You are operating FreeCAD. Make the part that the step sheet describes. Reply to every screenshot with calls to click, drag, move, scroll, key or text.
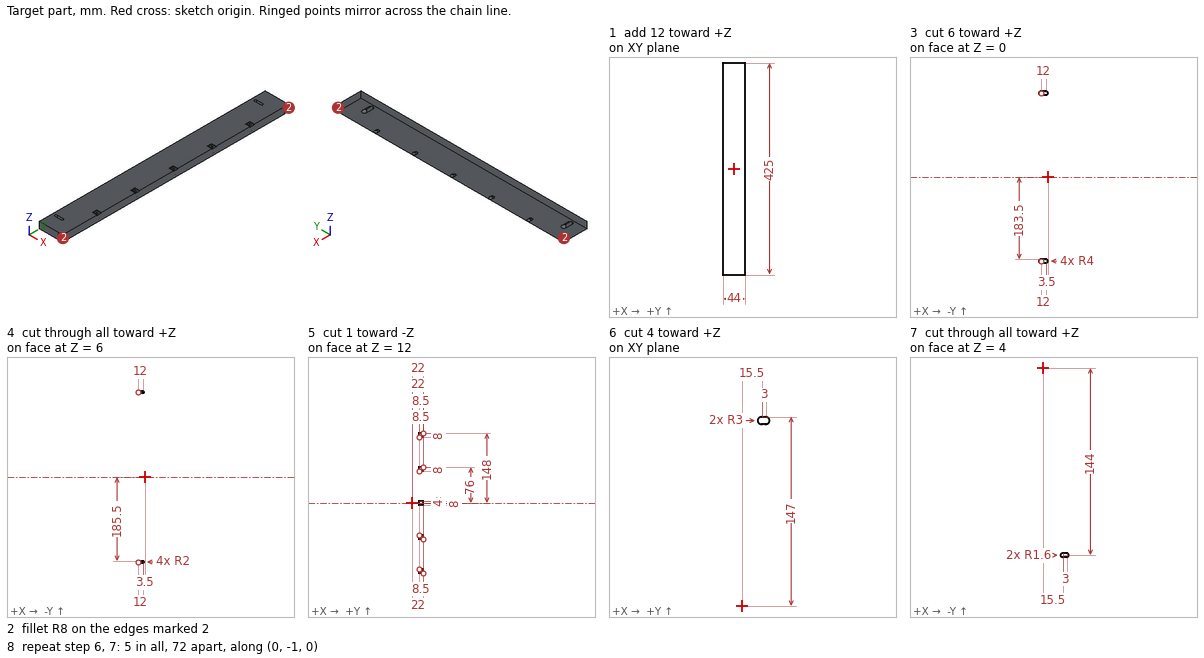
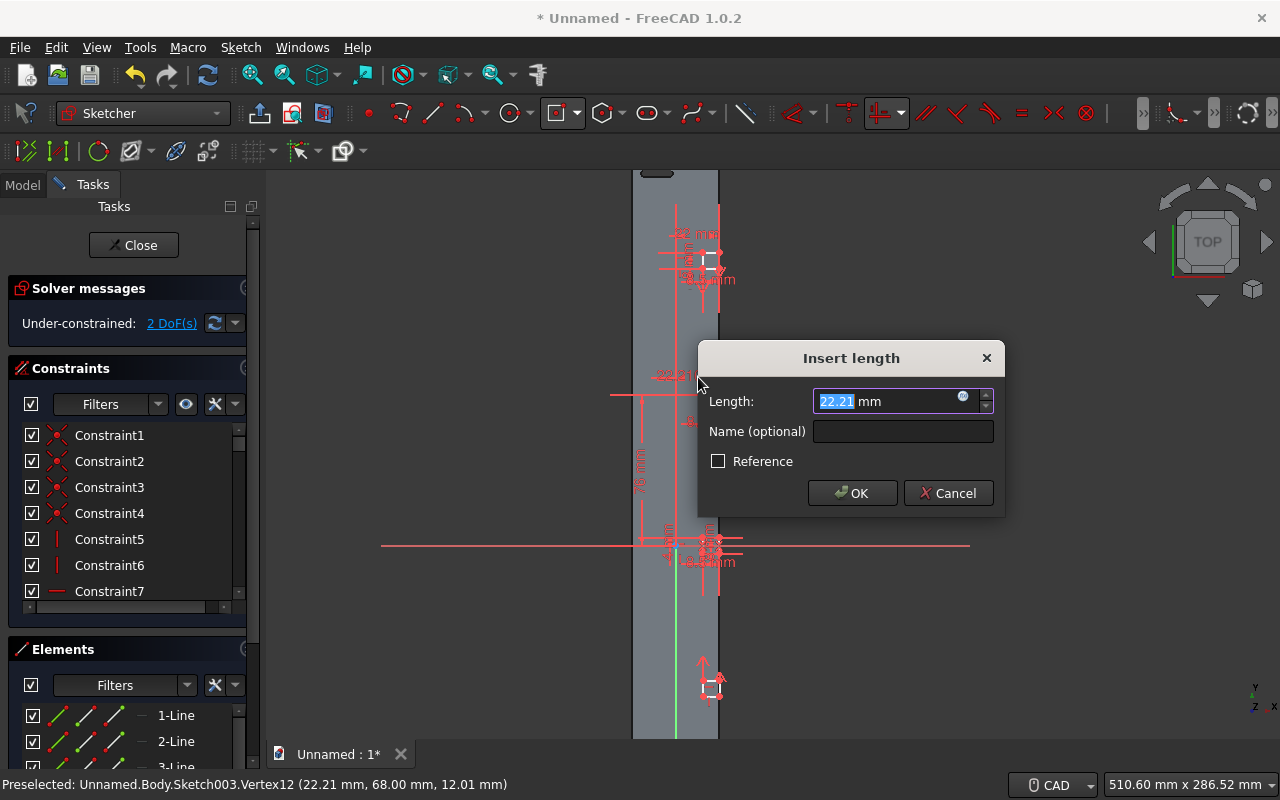
text(22)
key(Return)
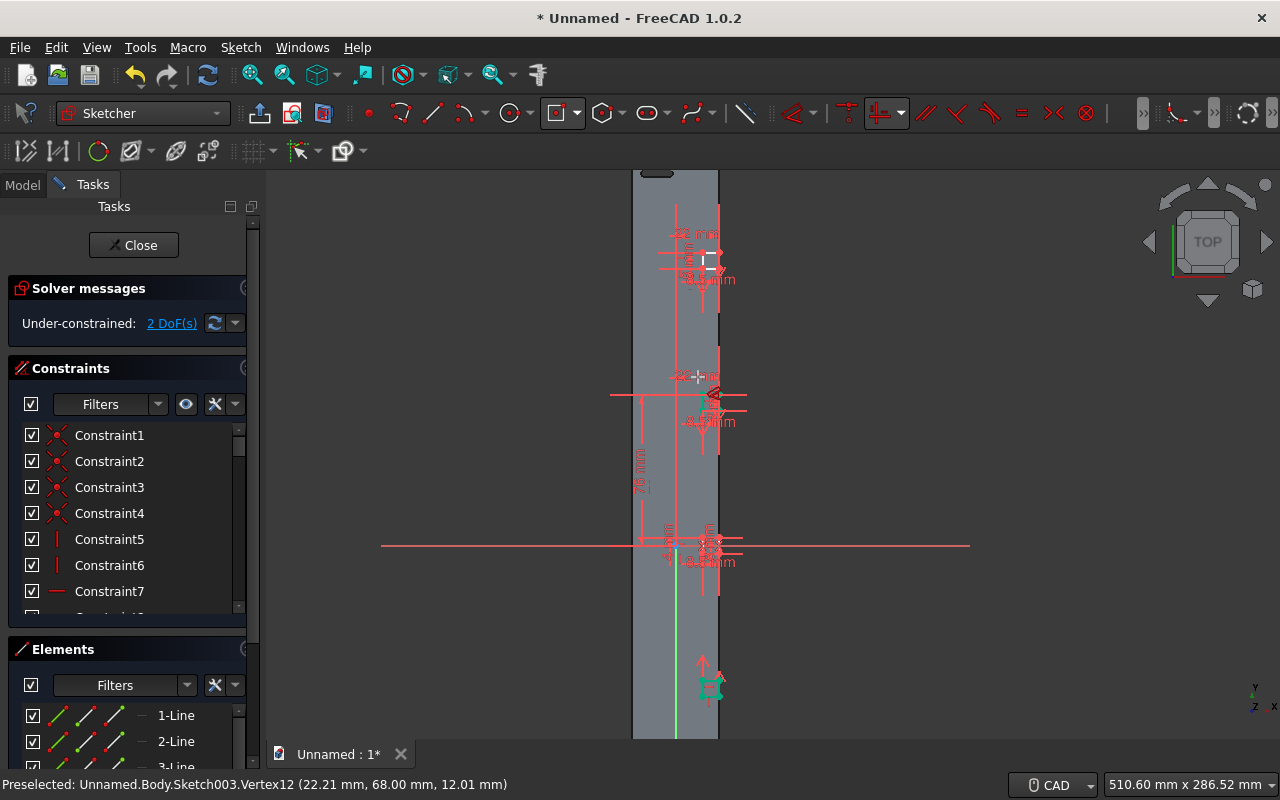
click(719, 554)
click(698, 588)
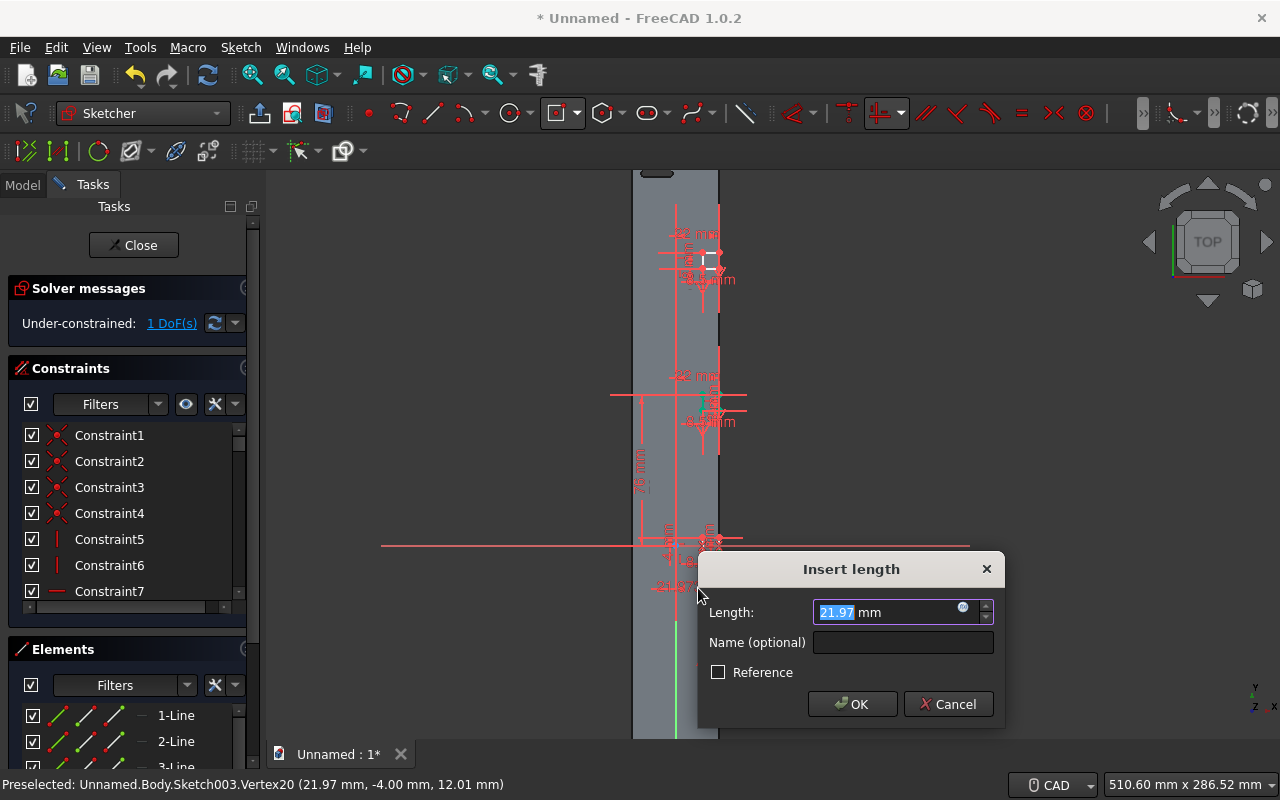
text(22)
key(Return)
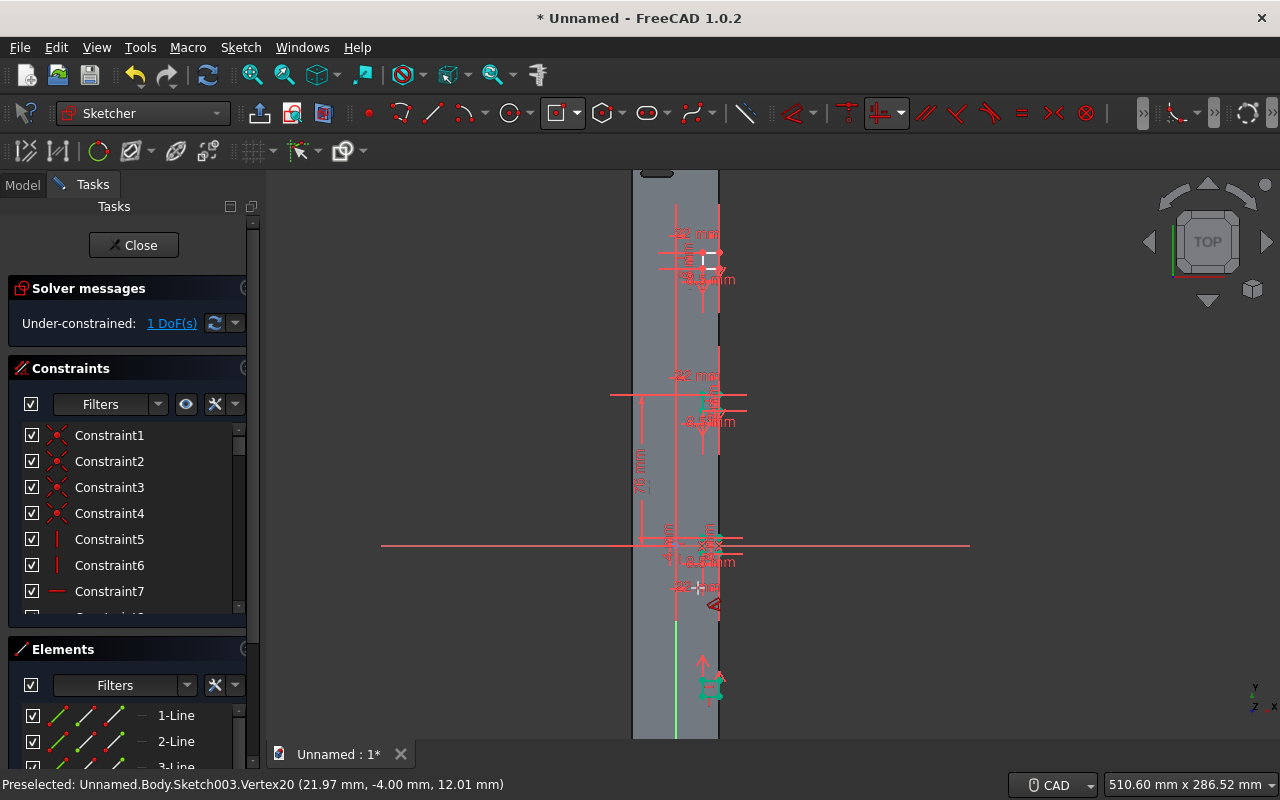
click(703, 253)
click(642, 399)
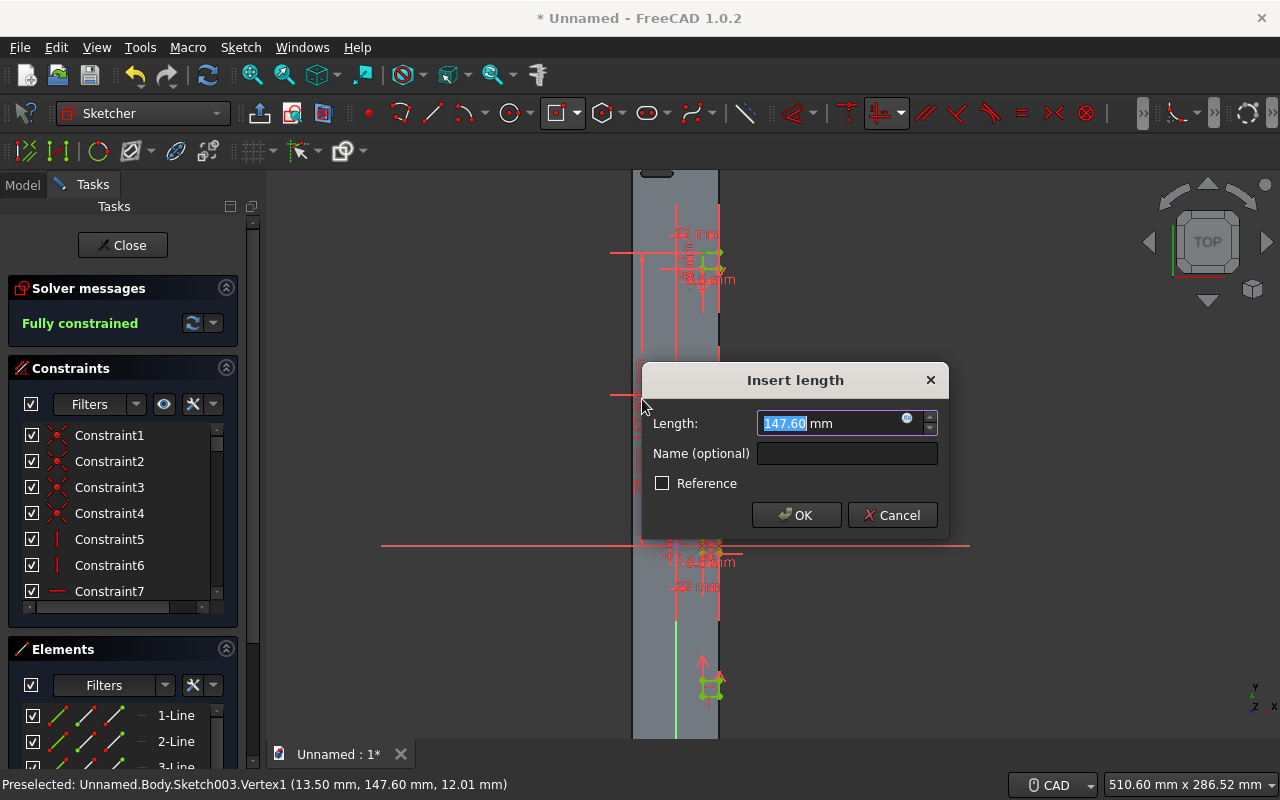
text(148)
key(Return)
key(Escape)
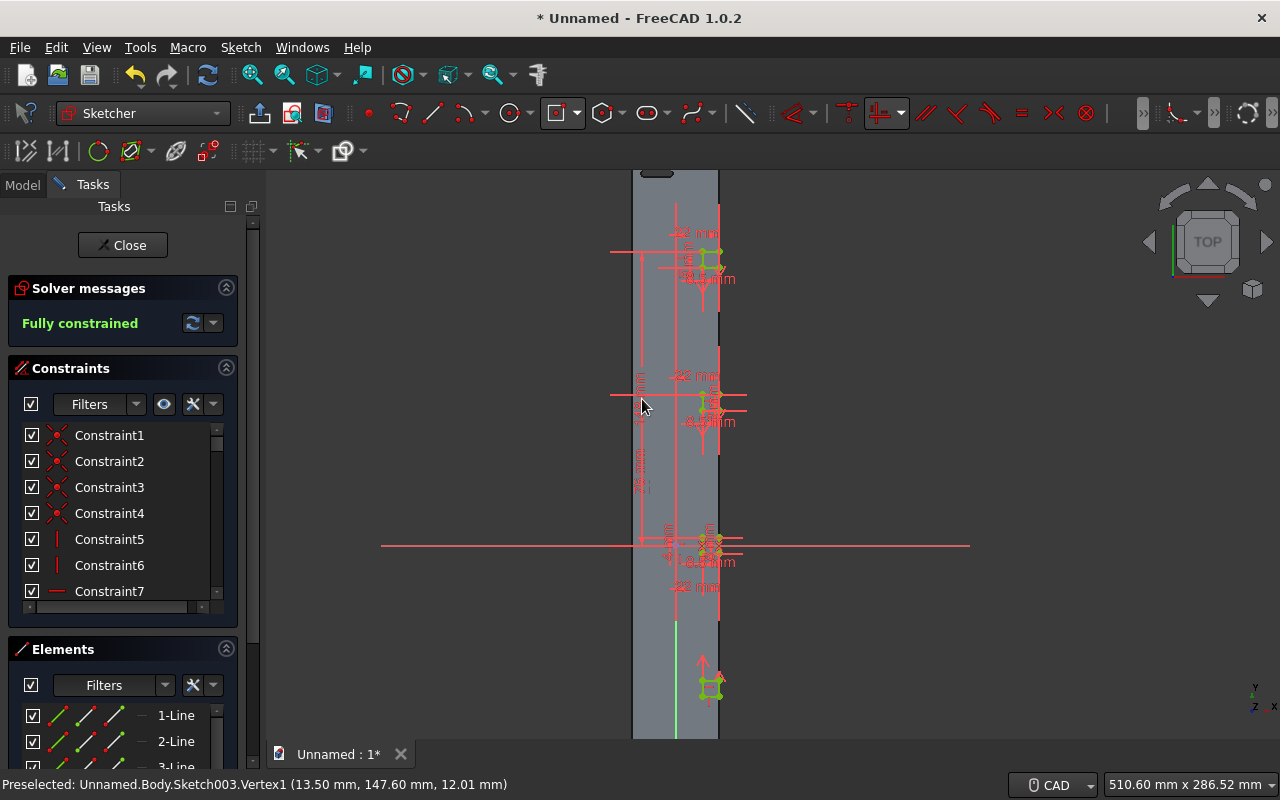
click(123, 245)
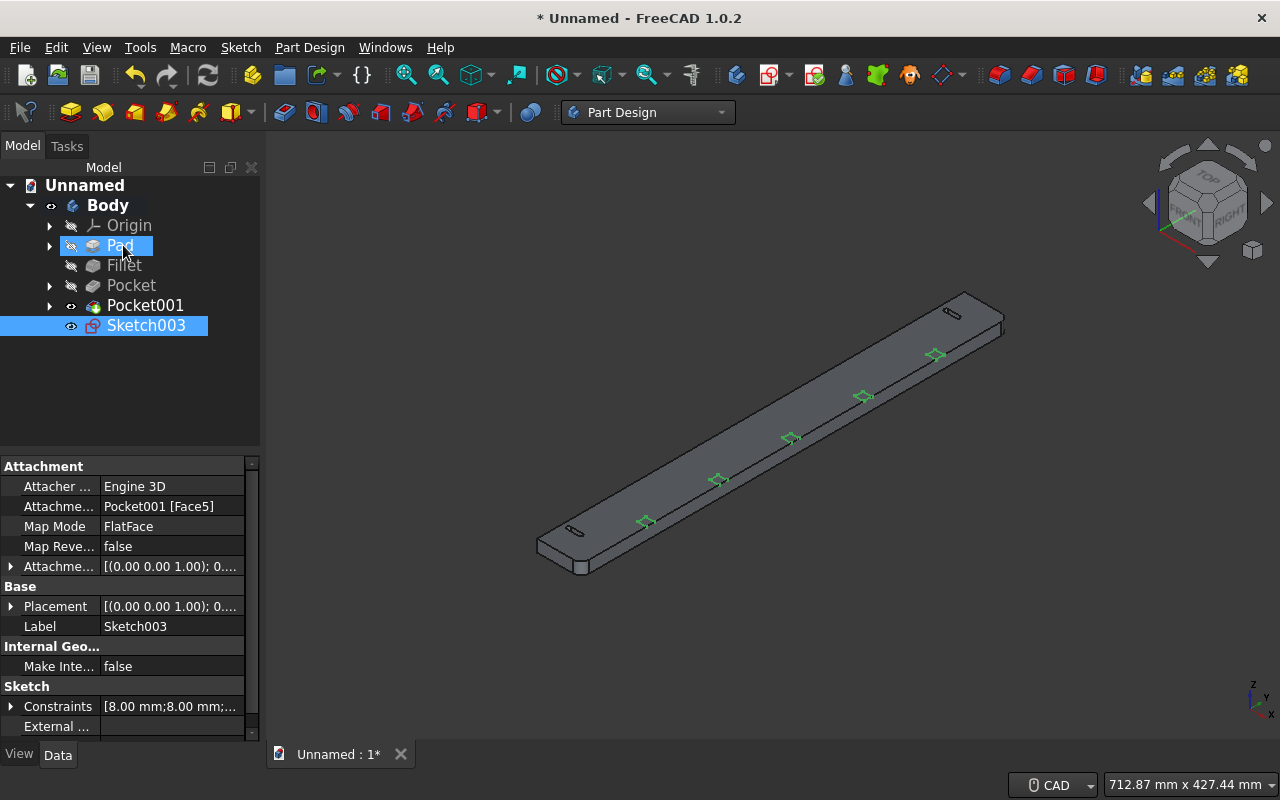
click(286, 112)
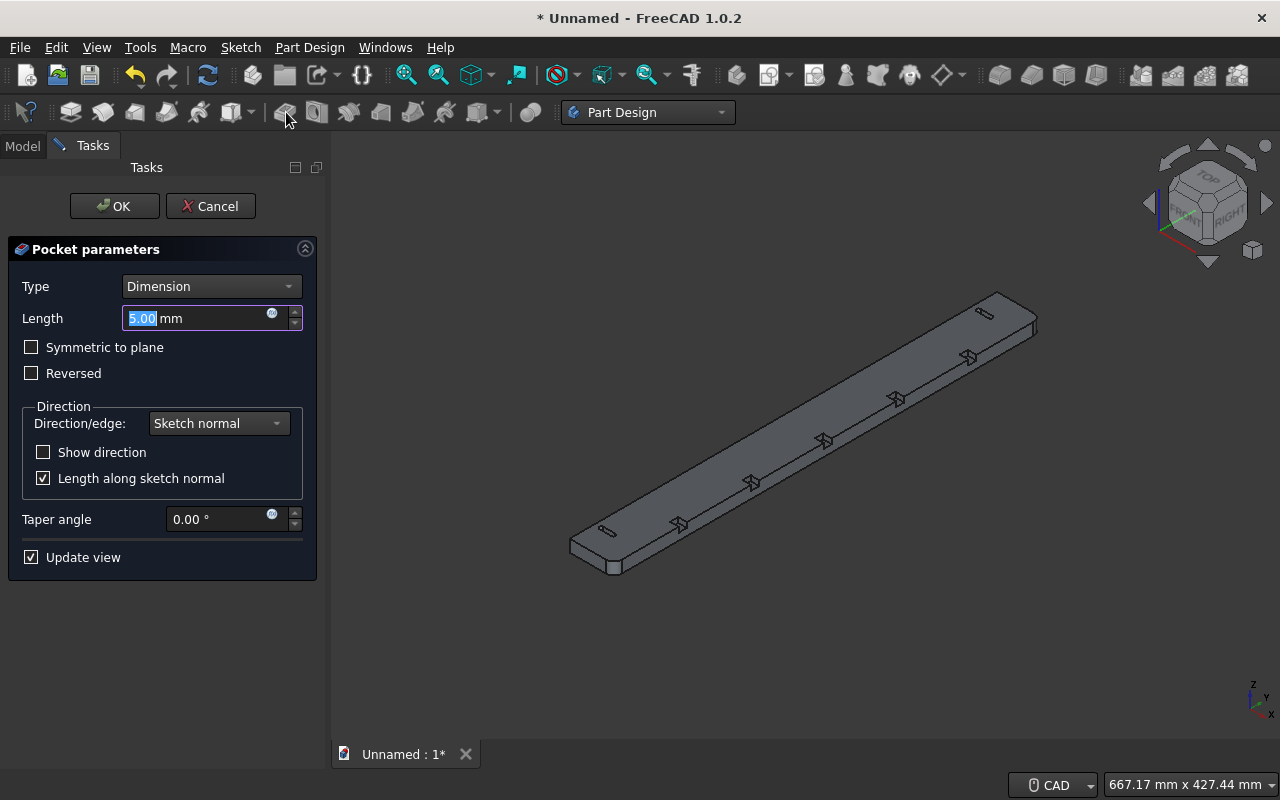
text(1)
key(Tab)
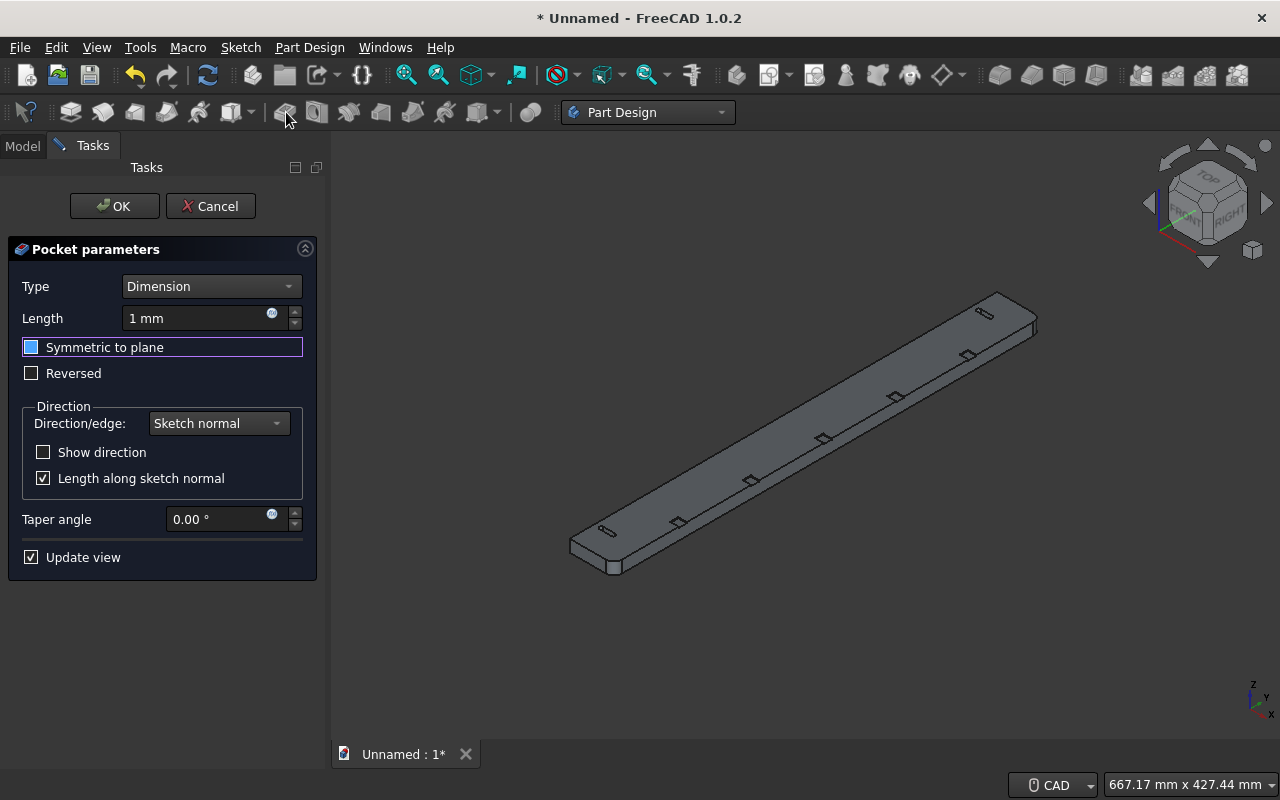
click(115, 206)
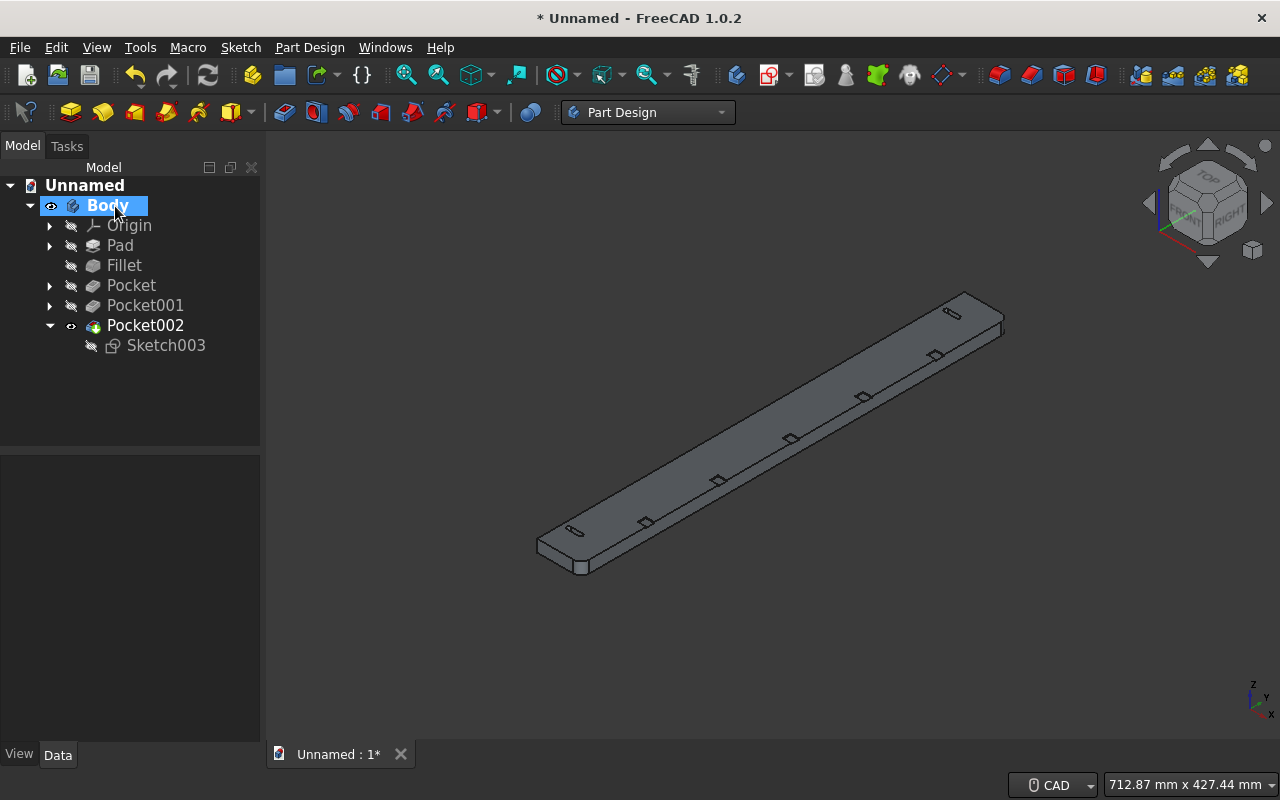
click(770, 76)